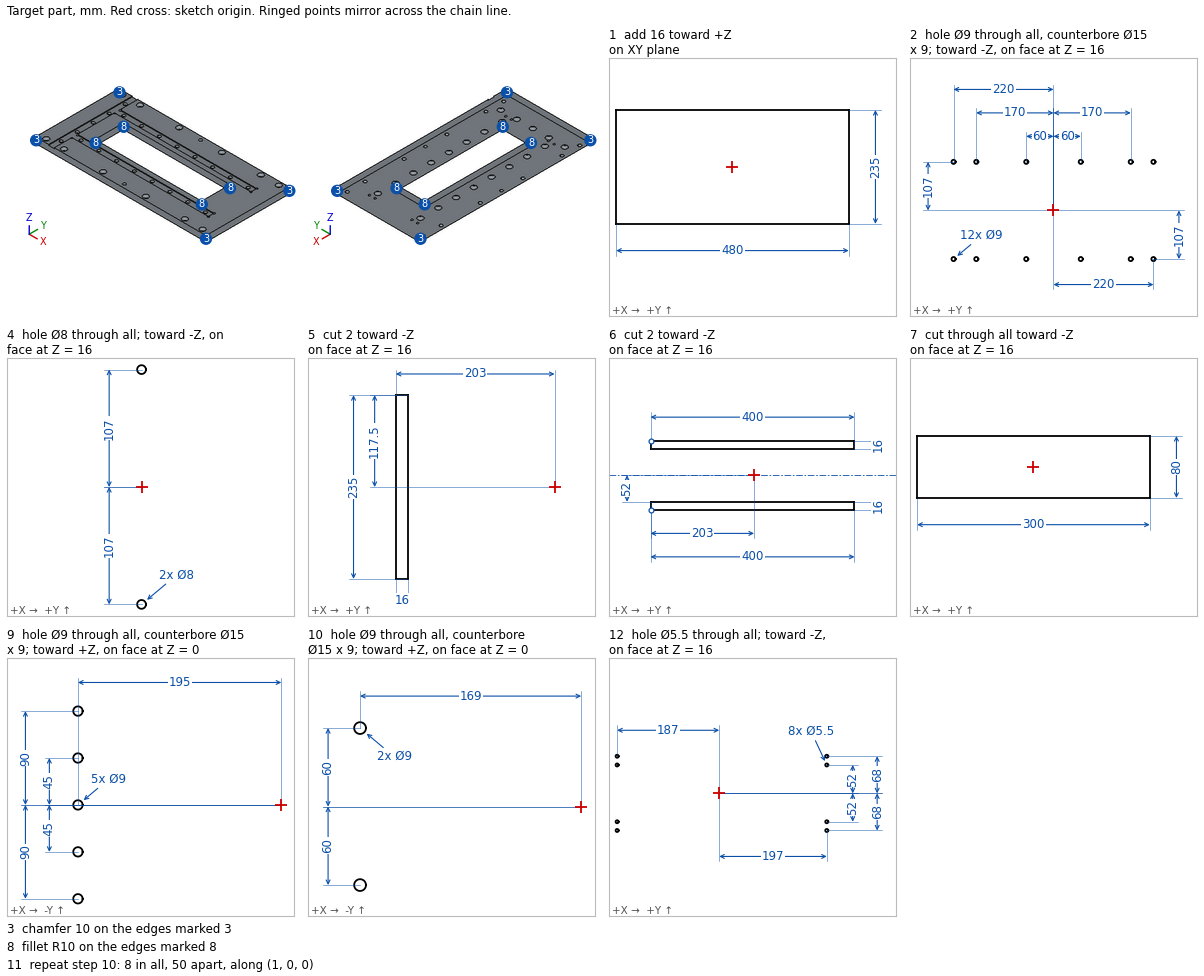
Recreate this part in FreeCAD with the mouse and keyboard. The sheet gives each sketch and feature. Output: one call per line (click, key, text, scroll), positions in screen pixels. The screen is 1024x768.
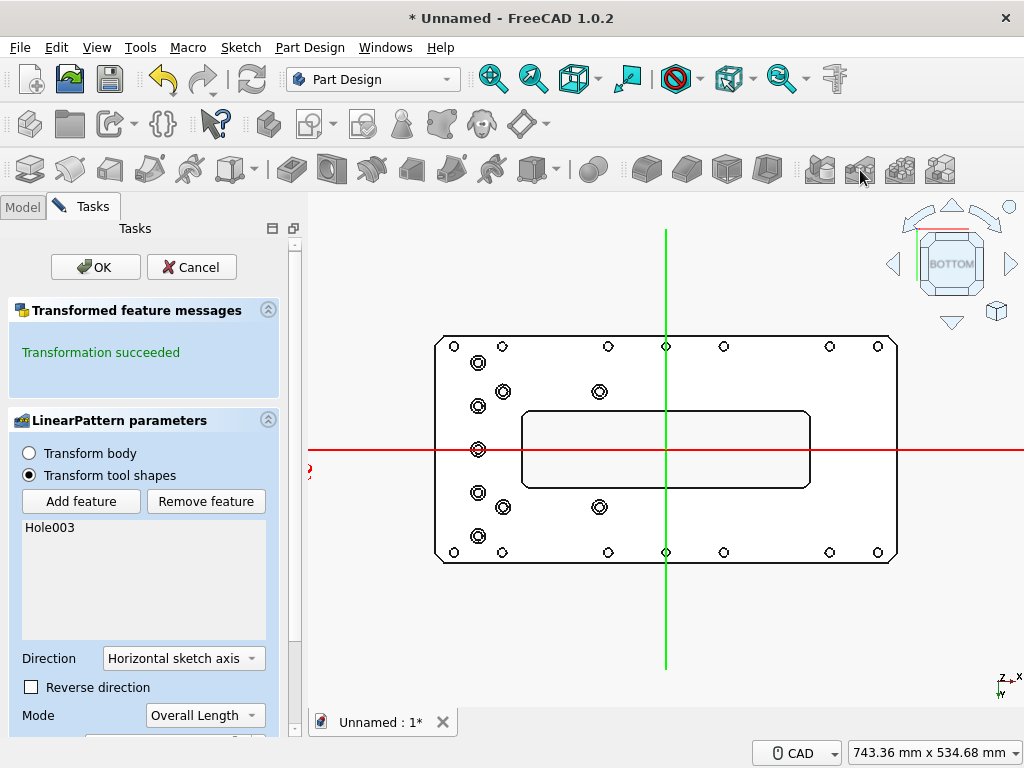
click(184, 658)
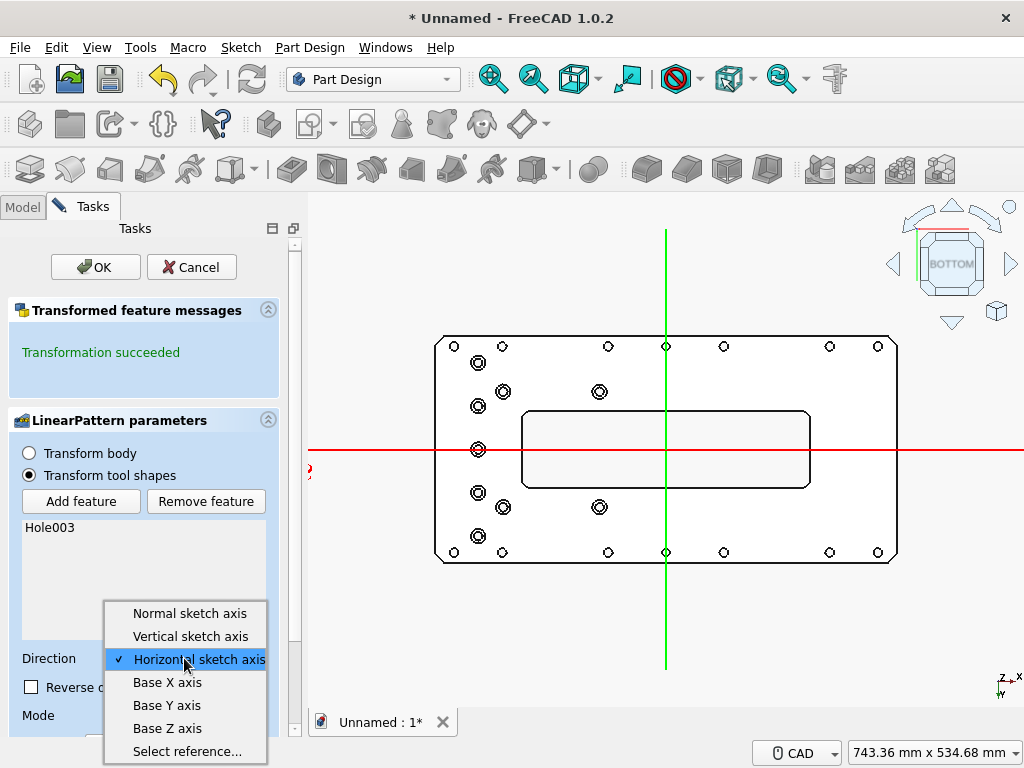
click(184, 682)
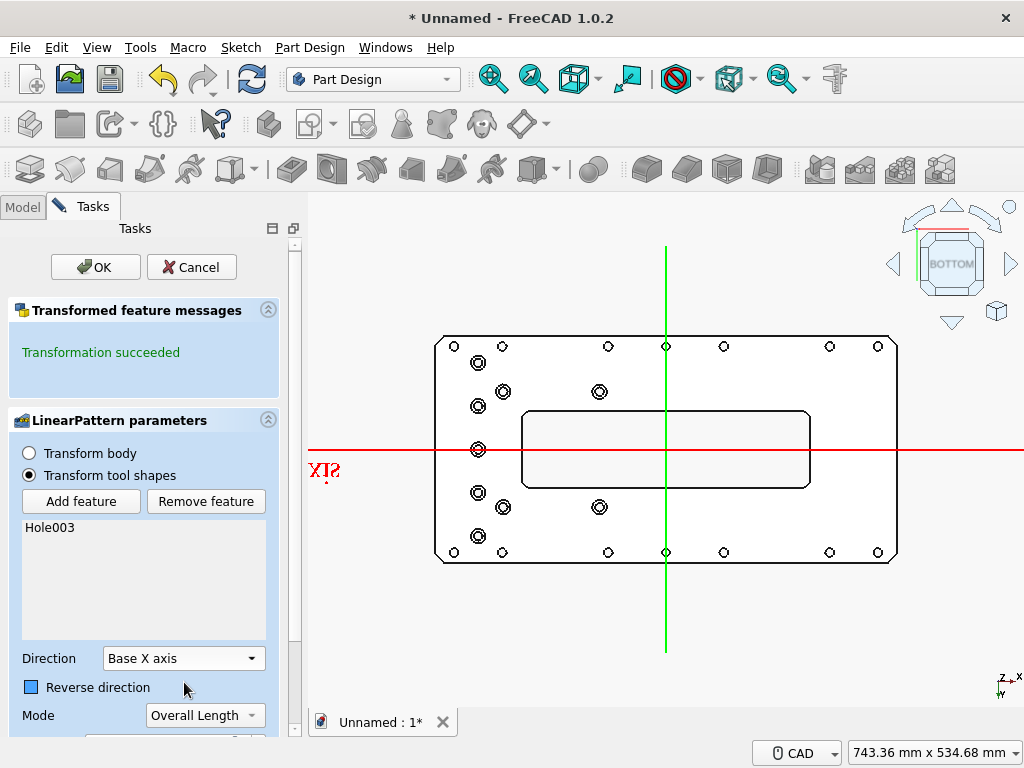
click(206, 716)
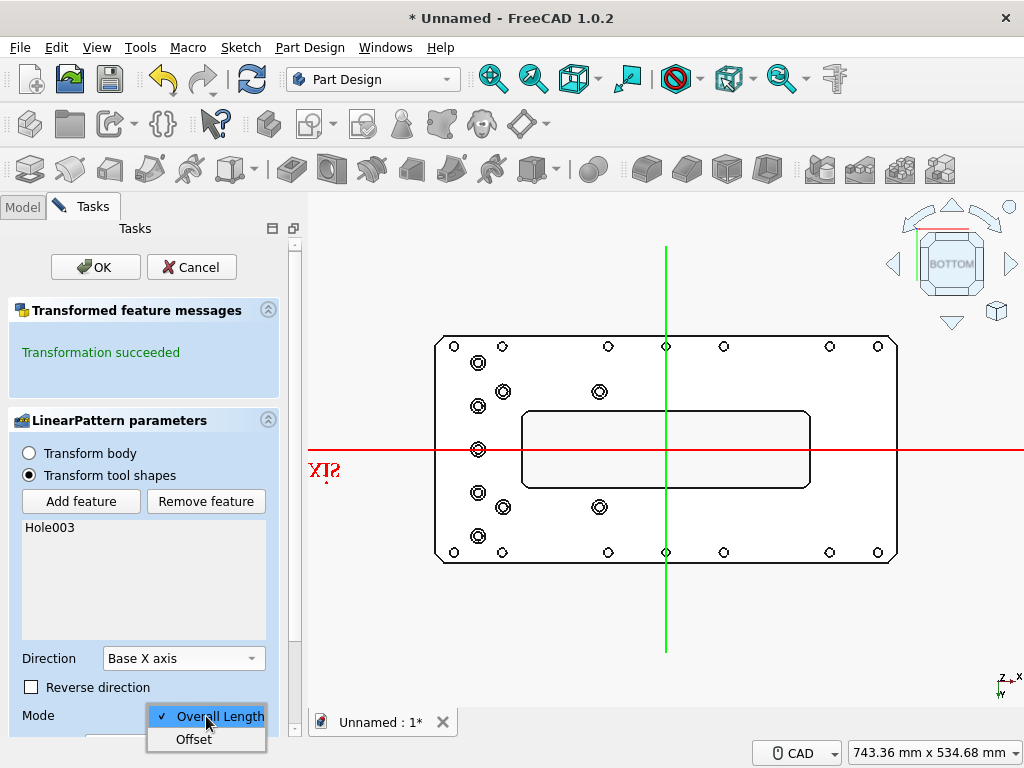
click(206, 740)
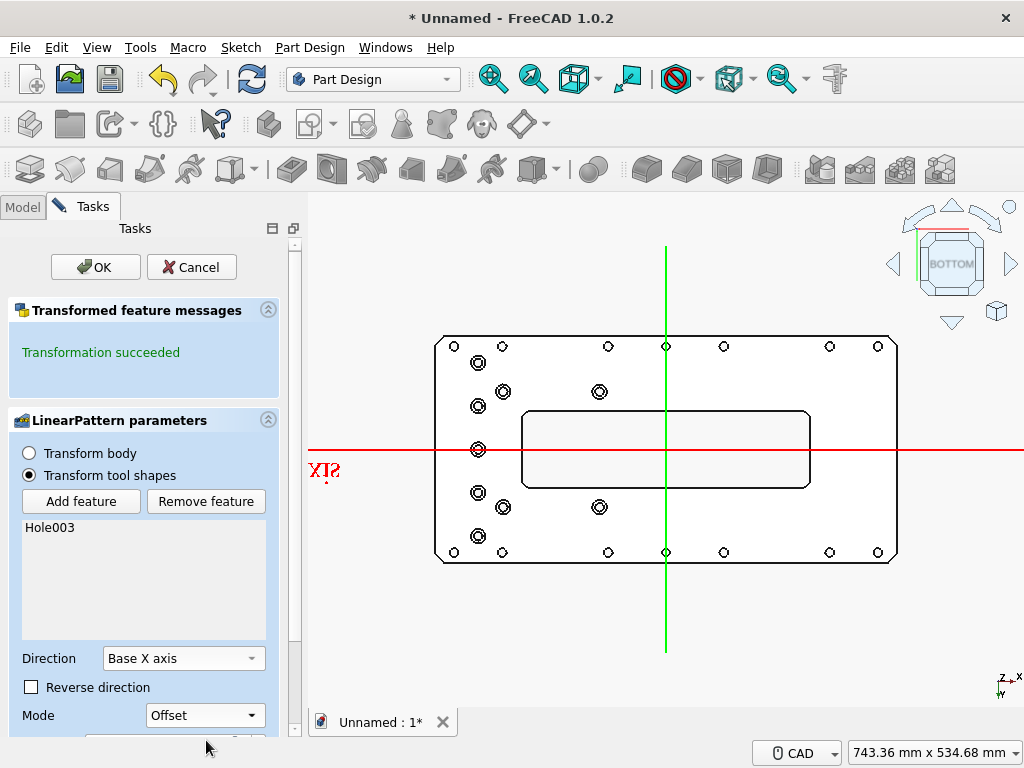
scroll(295, 487, down, 2)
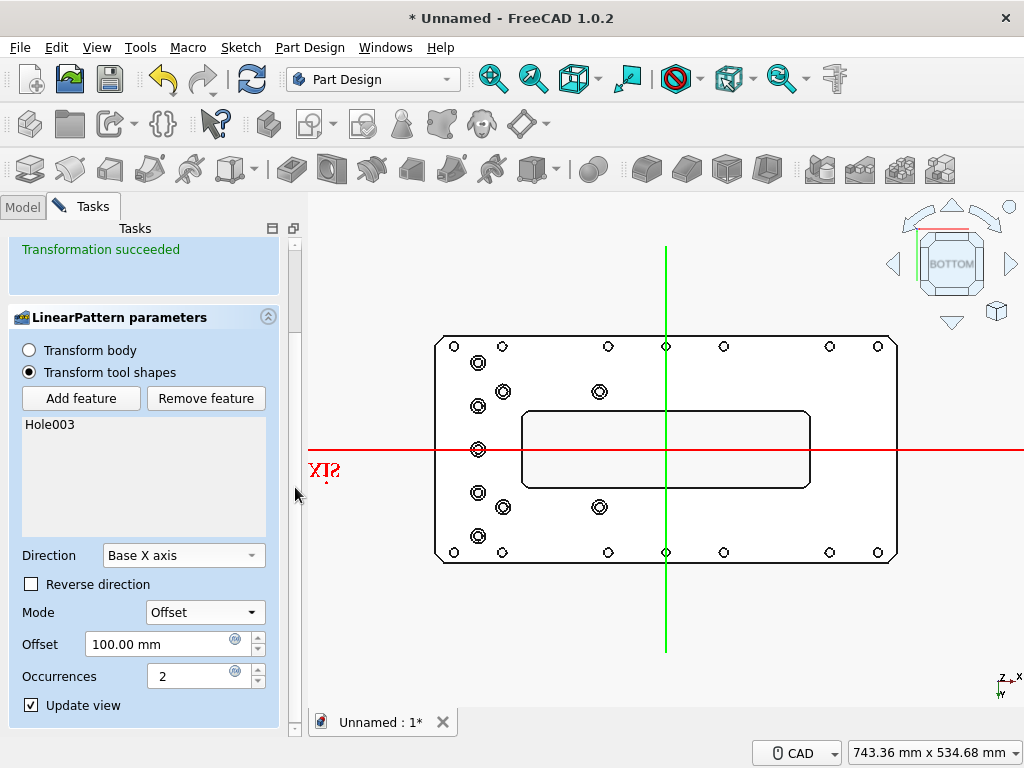
triple_click(168, 644)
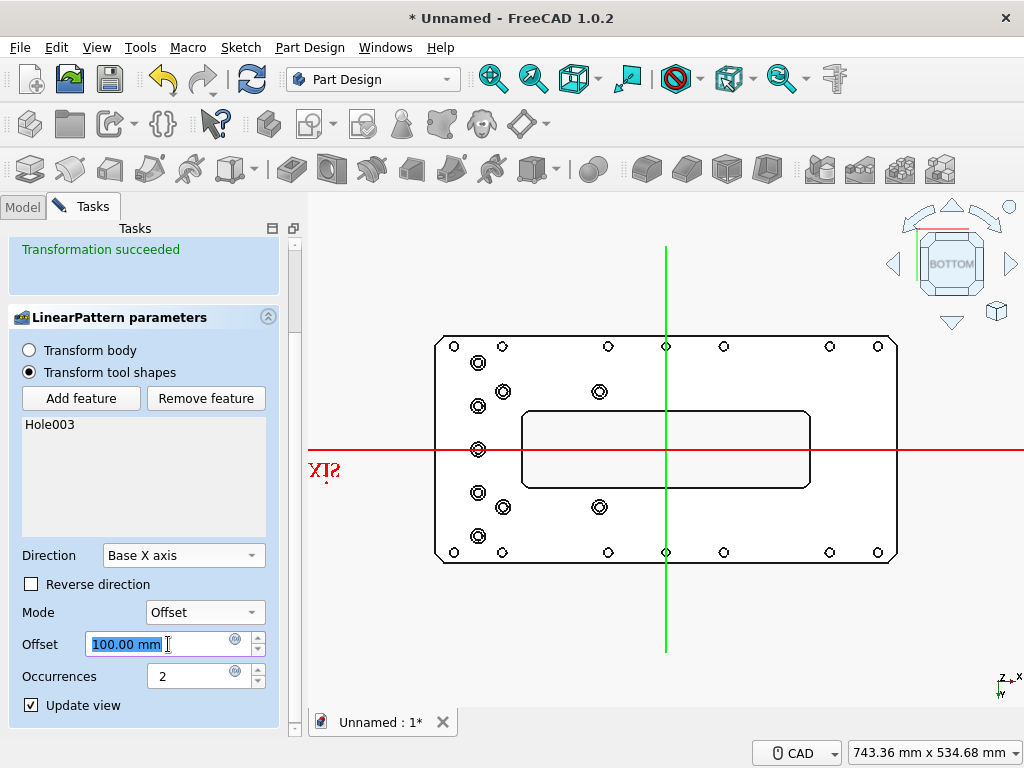
text(50)
key(Tab)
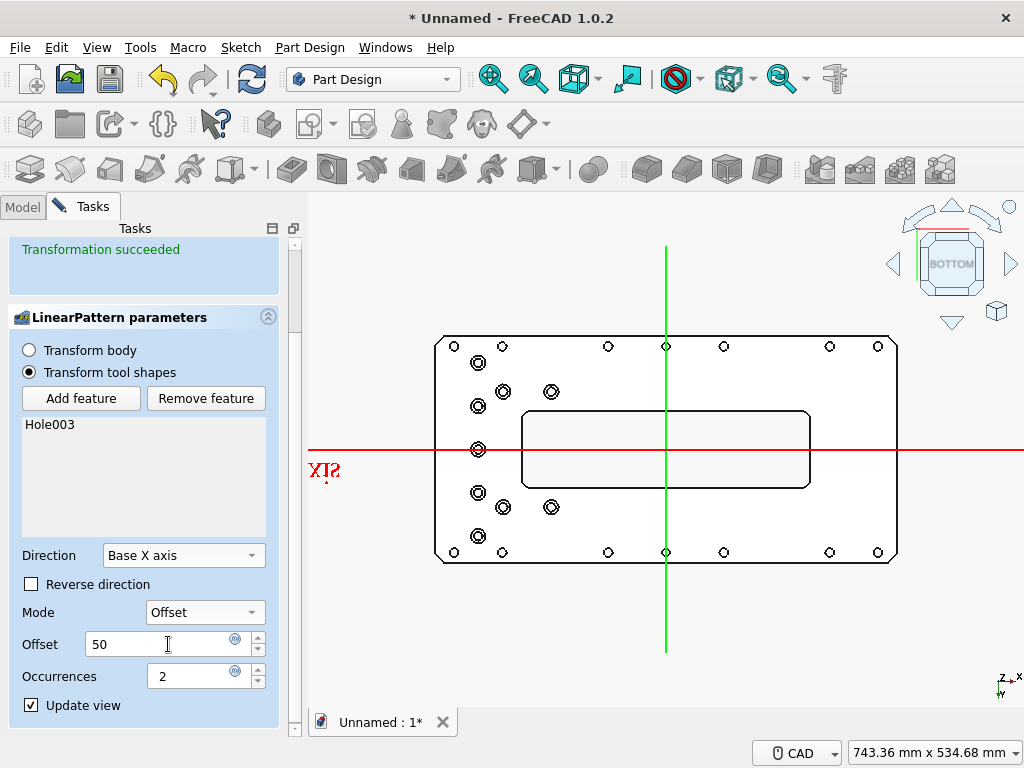
triple_click(198, 676)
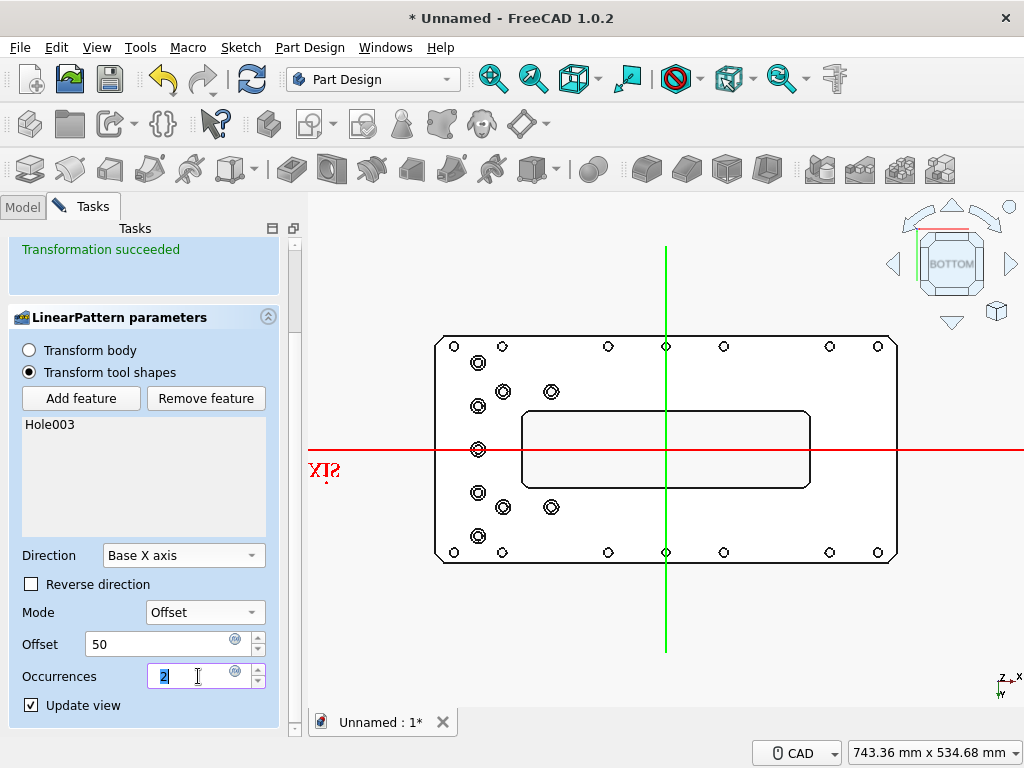
text(8)
key(Tab)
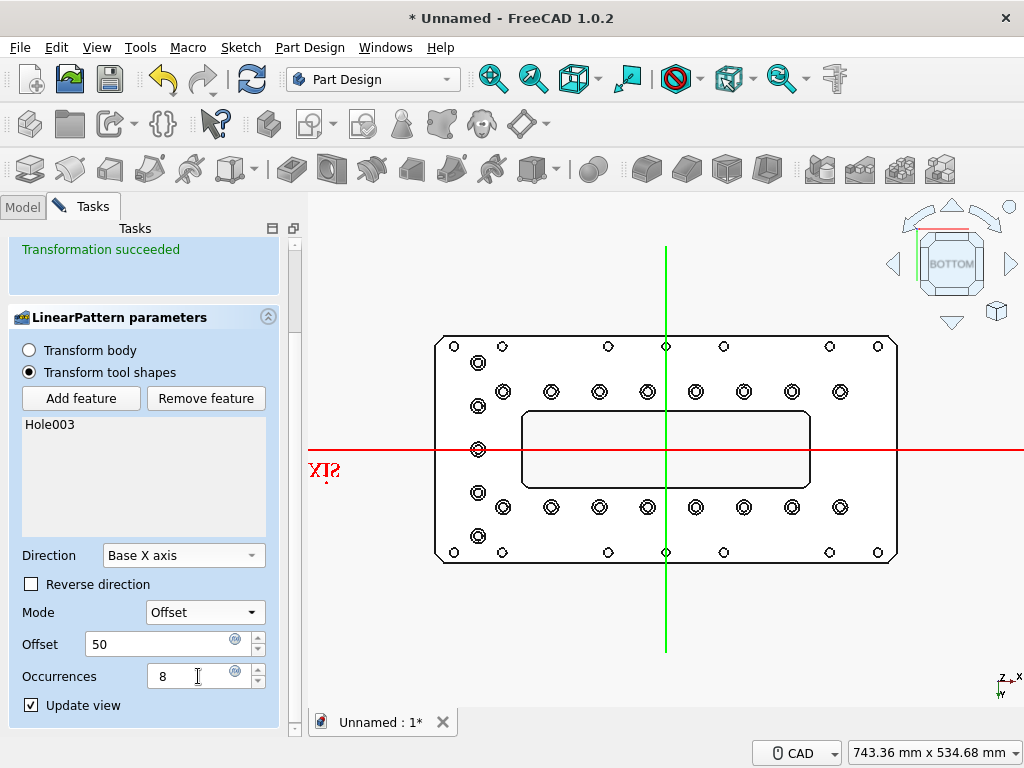
scroll(295, 487, up, 3)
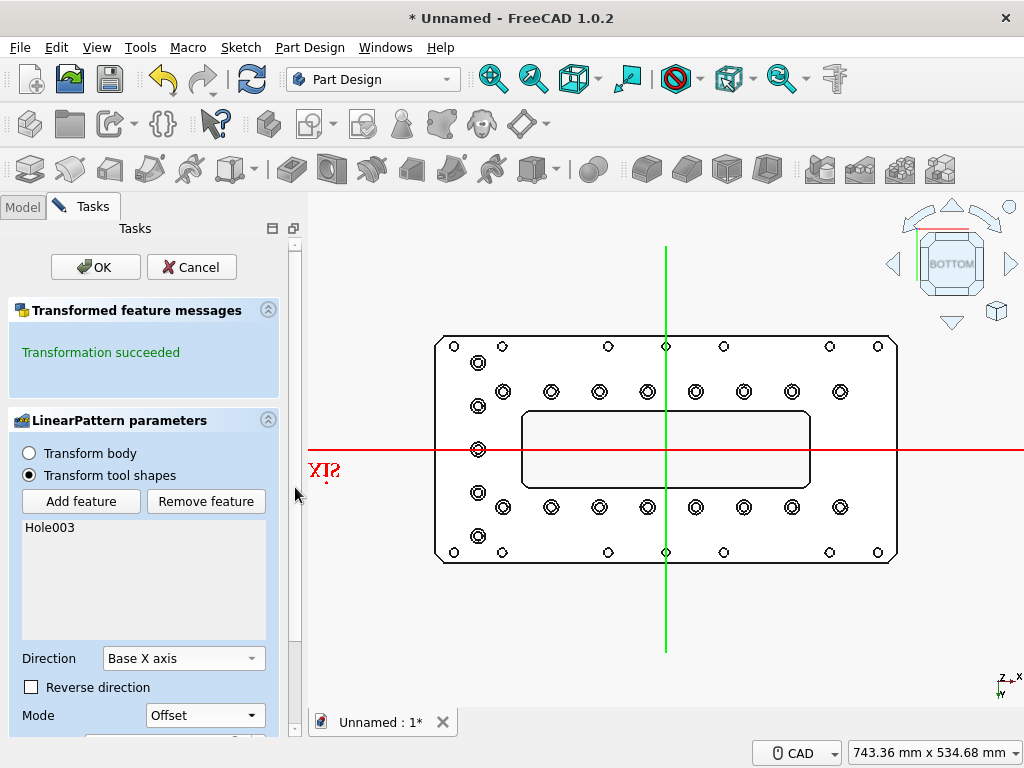
click(96, 267)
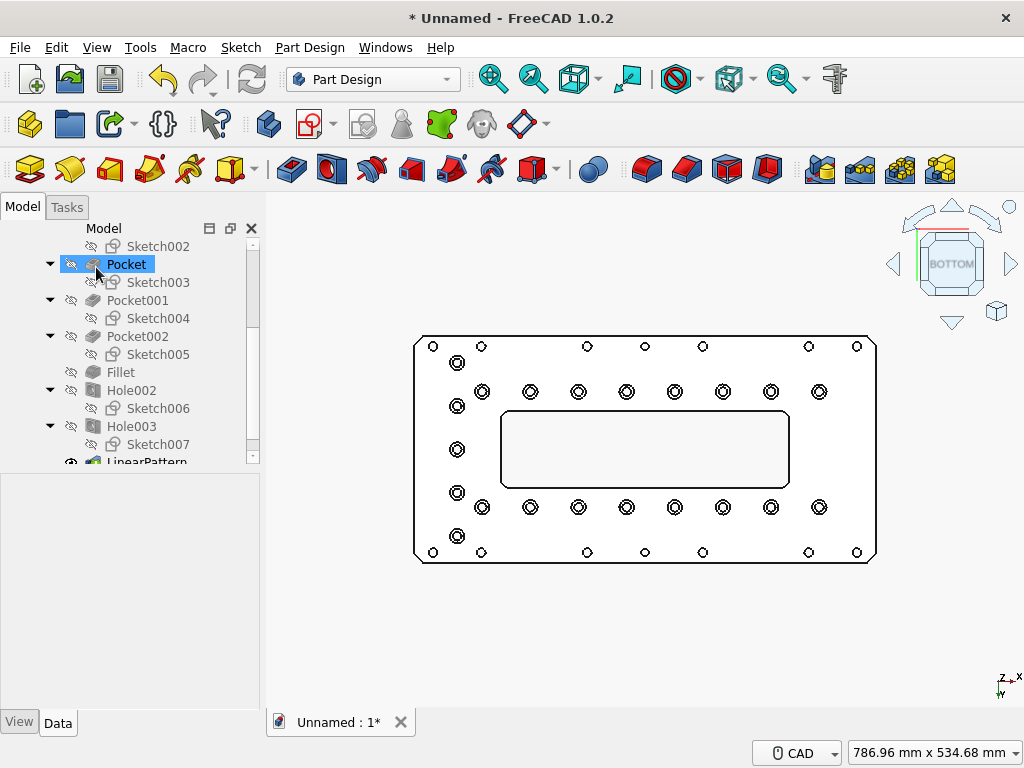
key(0)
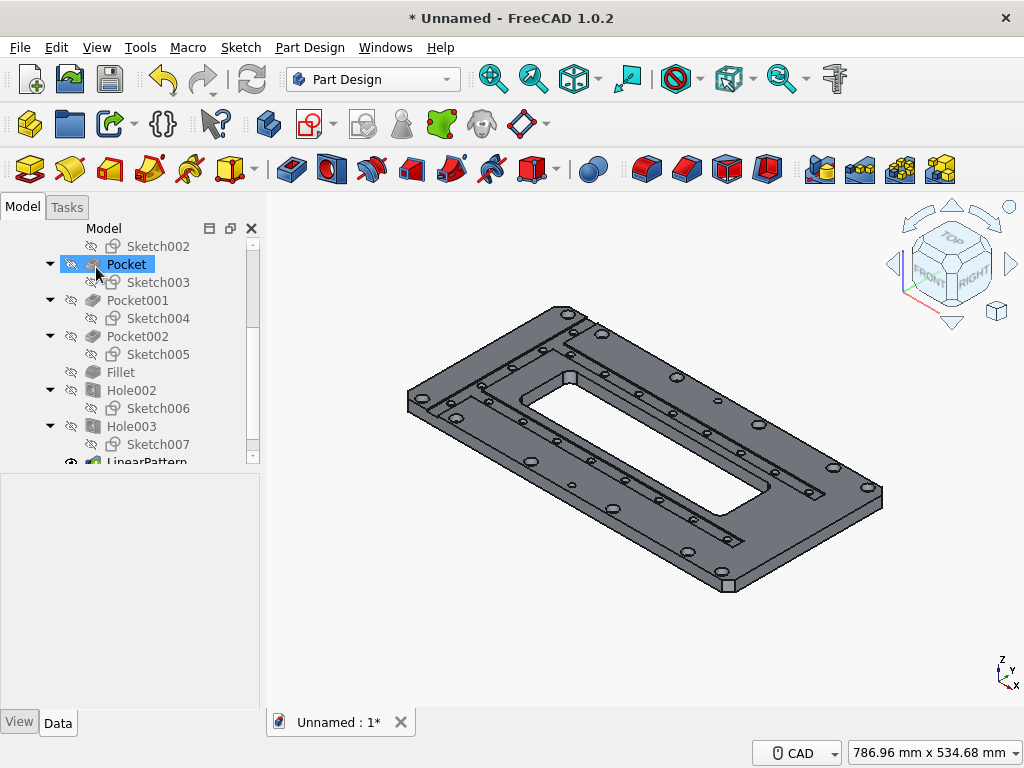
click(788, 525)